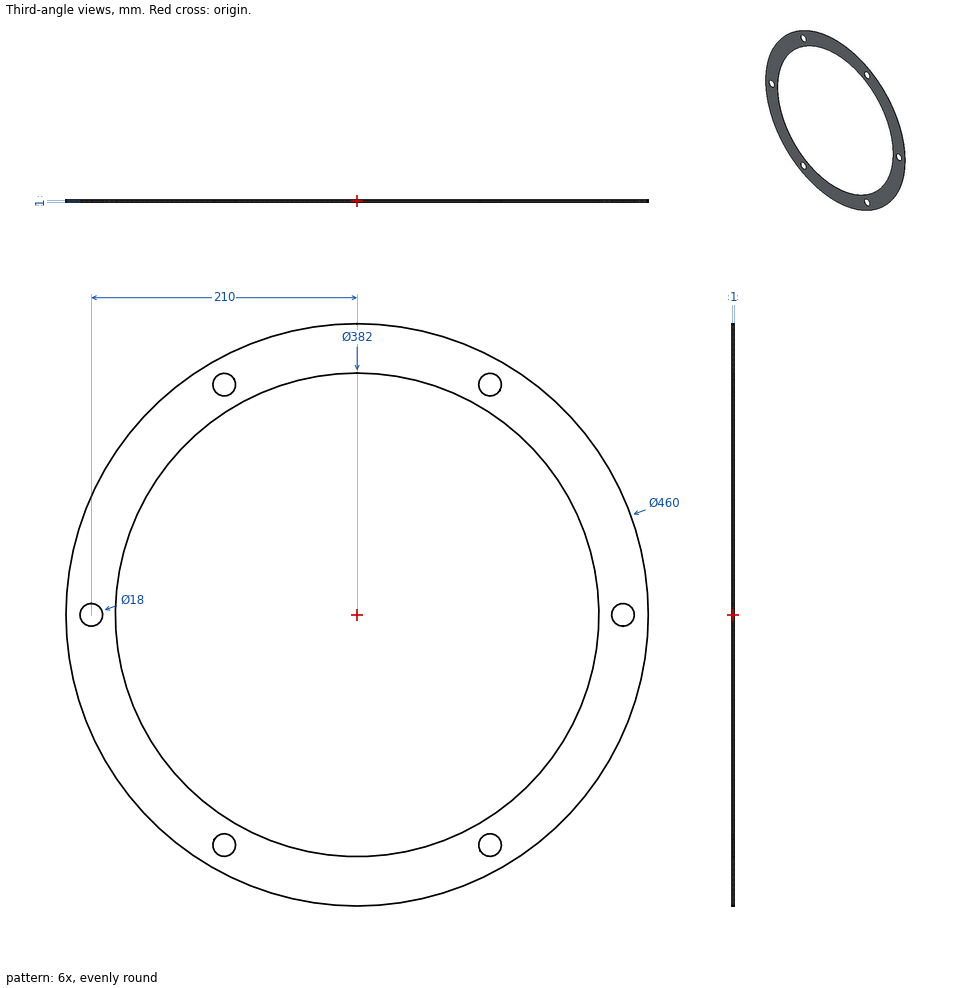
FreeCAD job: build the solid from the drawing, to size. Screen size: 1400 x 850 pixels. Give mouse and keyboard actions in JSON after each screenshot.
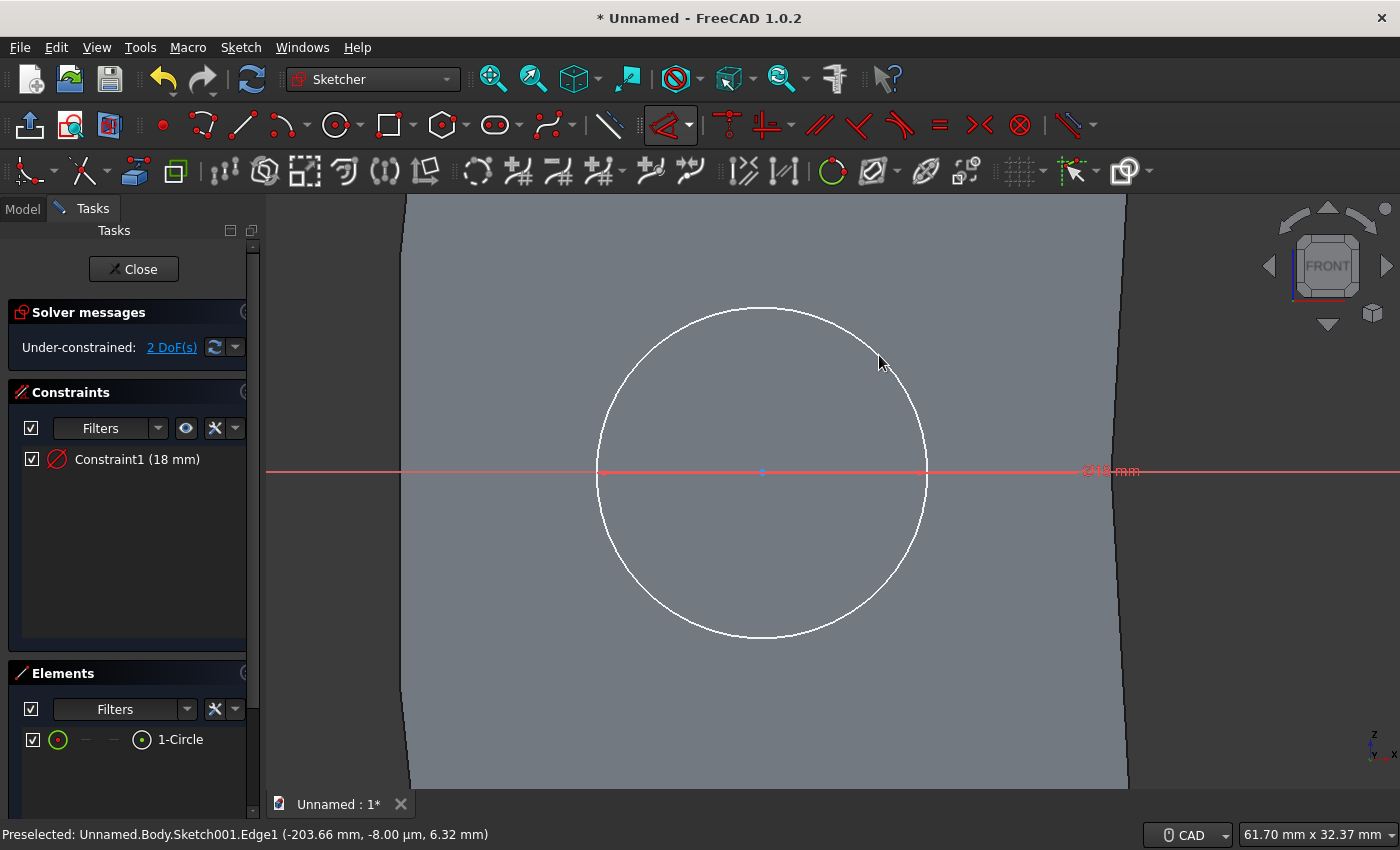
{"action": "left_click", "coordinate": [762, 473]}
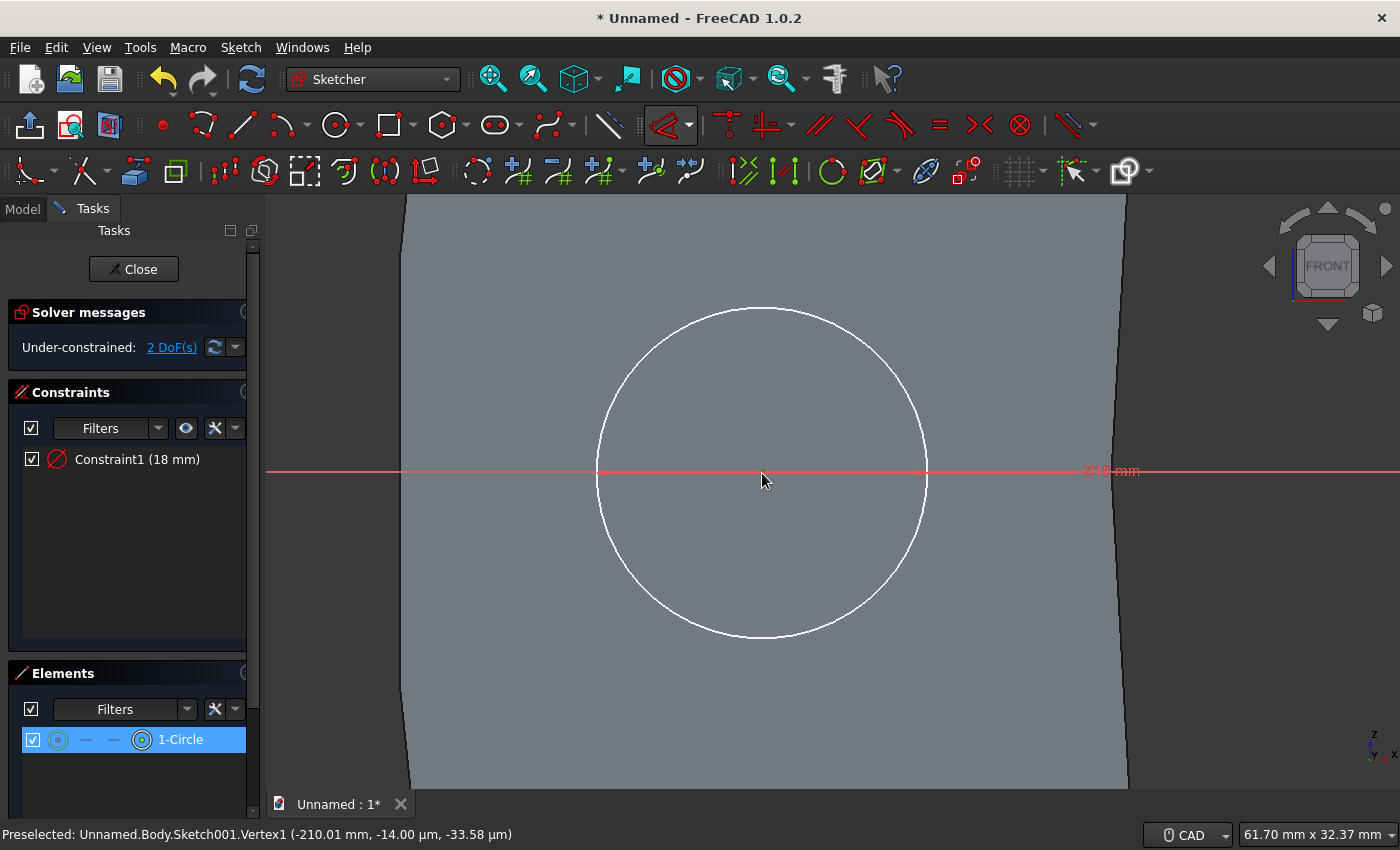
{"action": "left_click", "coordinate": [361, 472]}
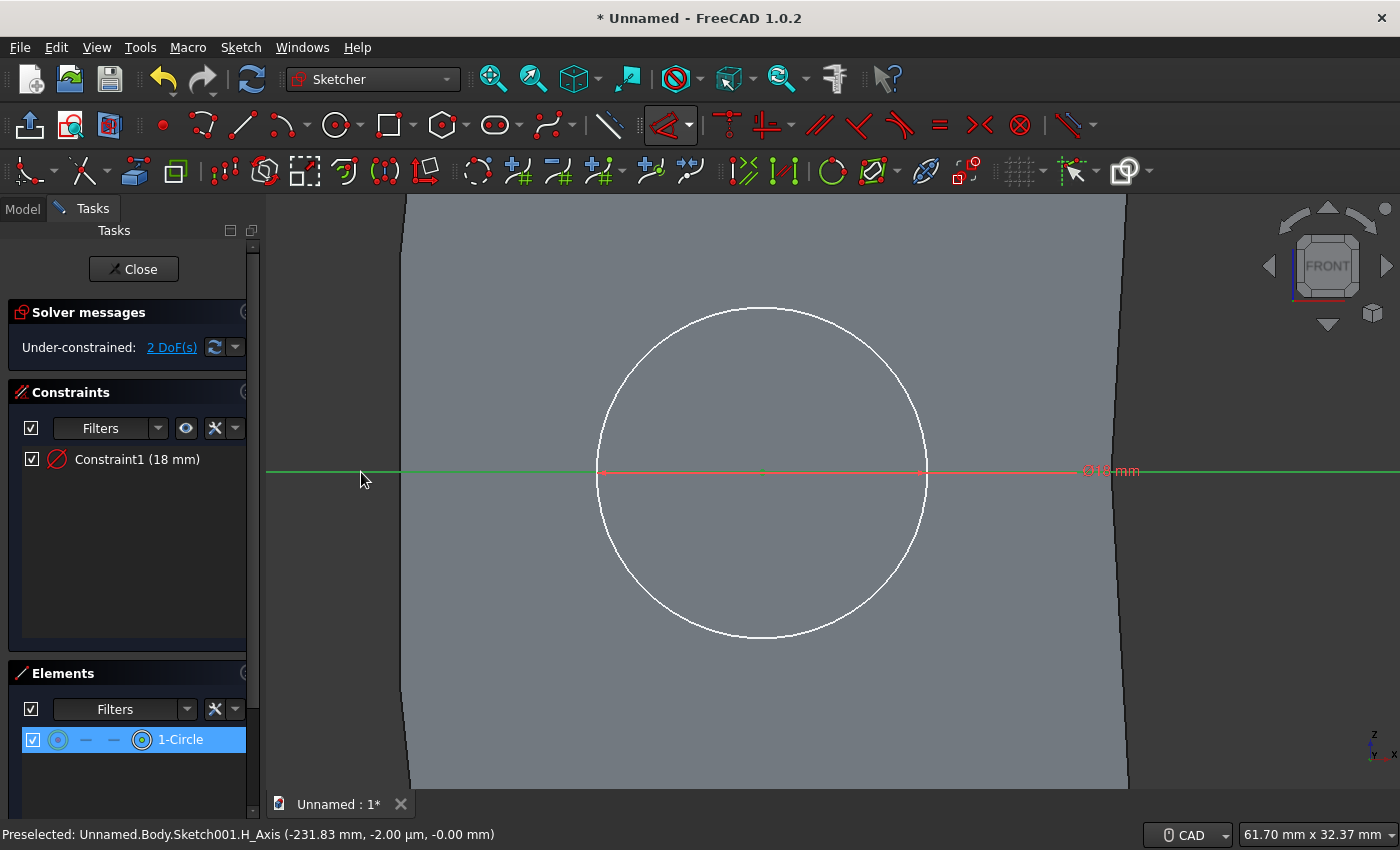
{"action": "left_click", "coordinate": [728, 126]}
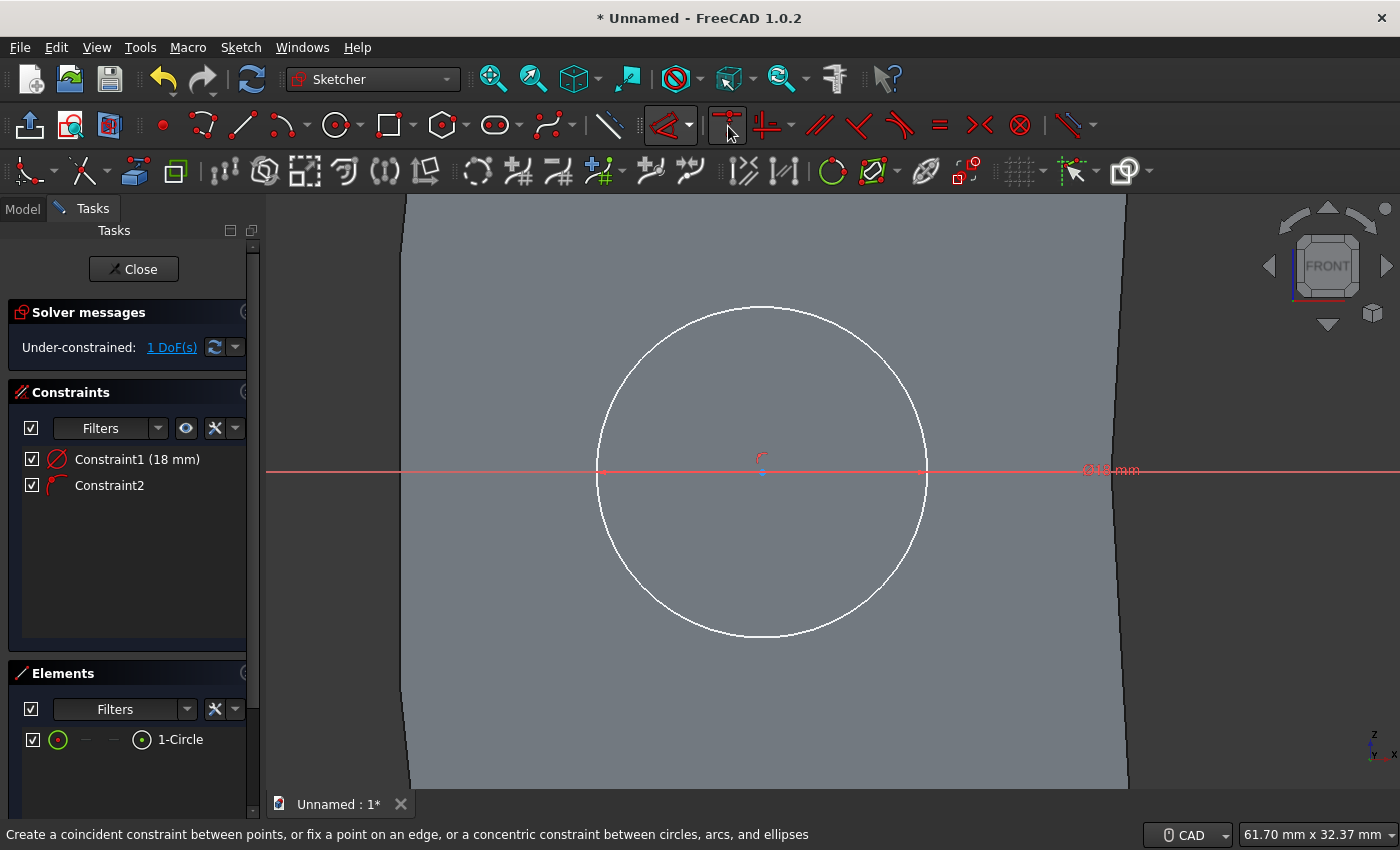
{"action": "left_click", "coordinate": [762, 472]}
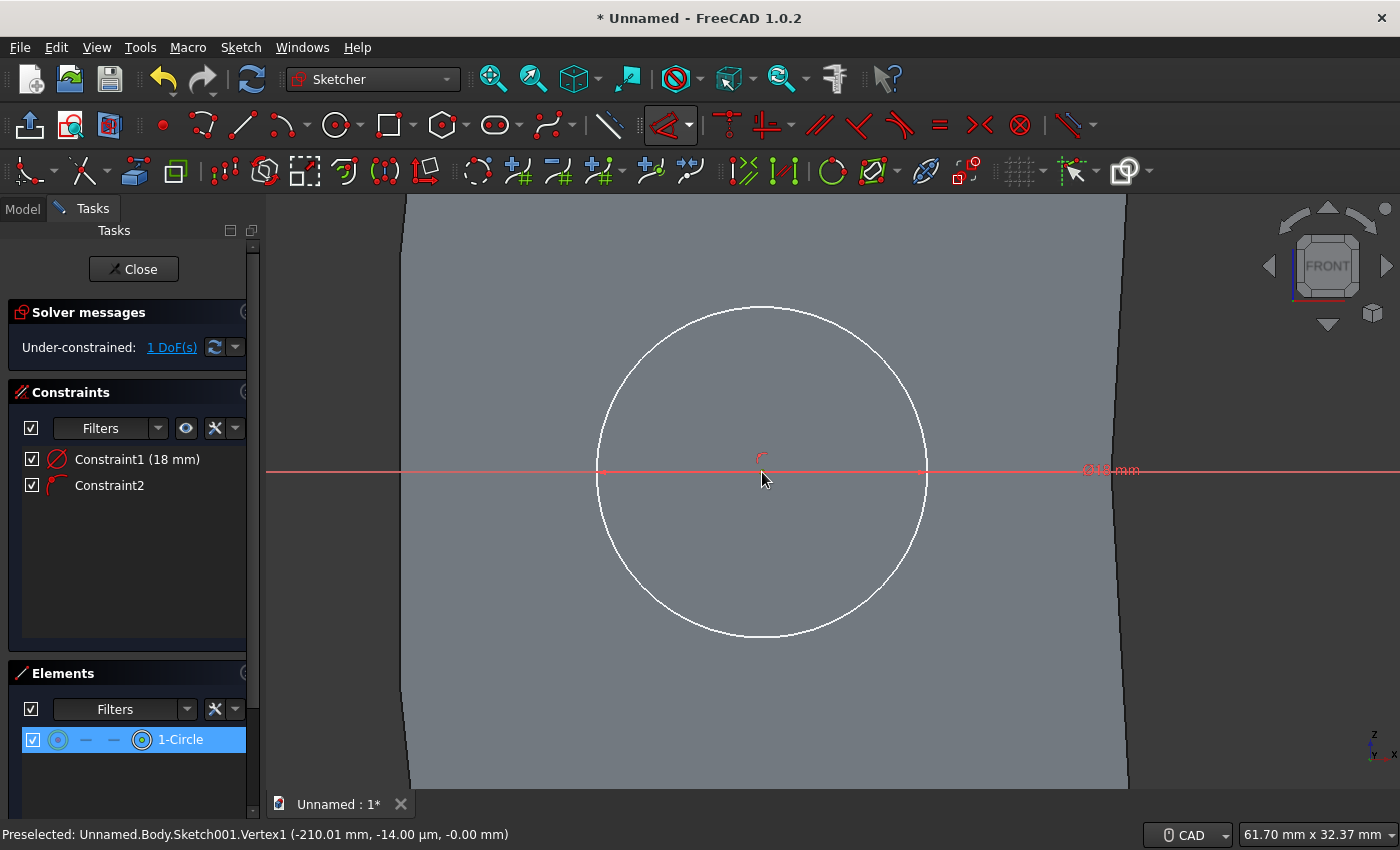
{"action": "key", "text": "l"}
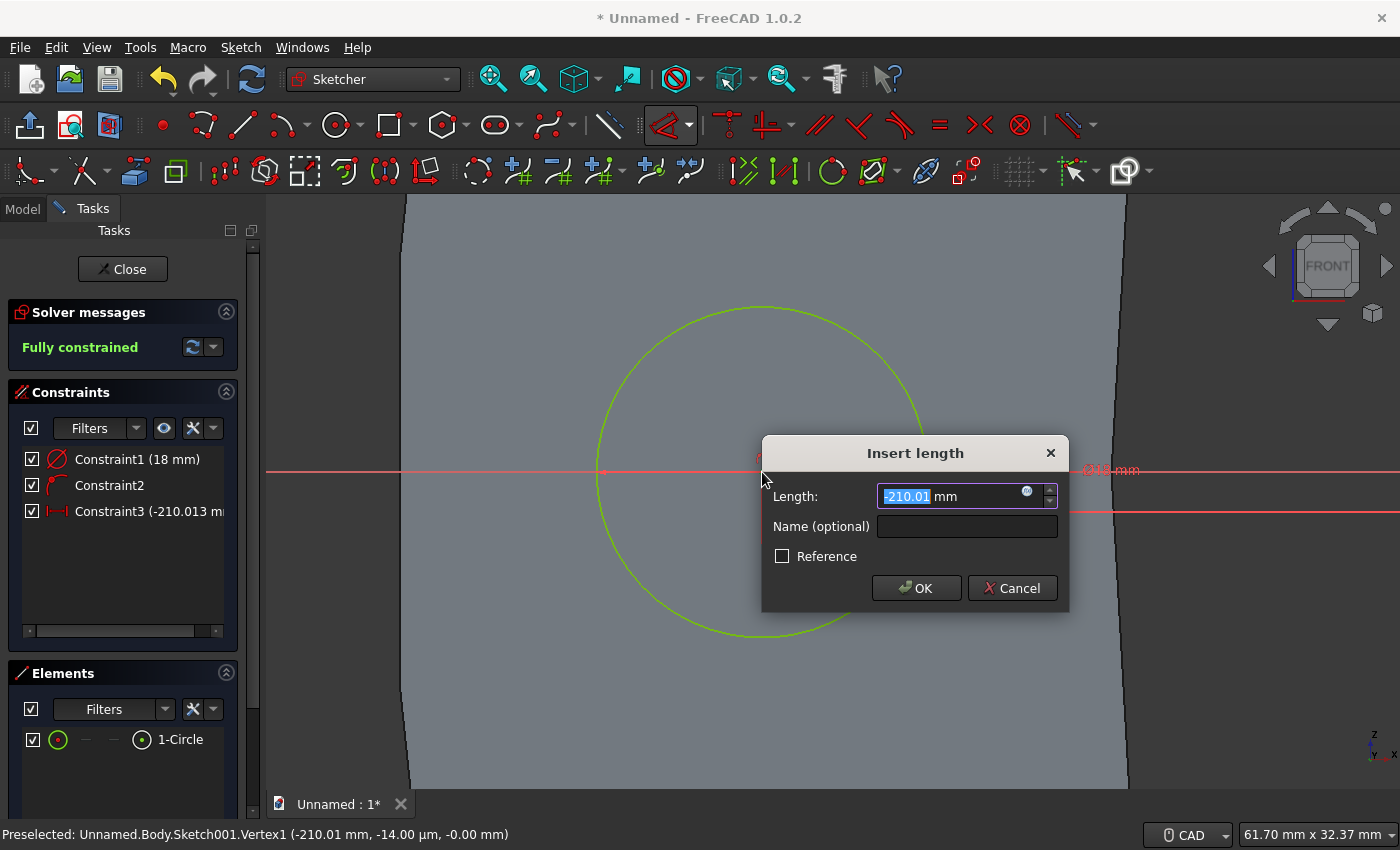
{"action": "type", "text": "-210"}
{"action": "key", "text": "Return"}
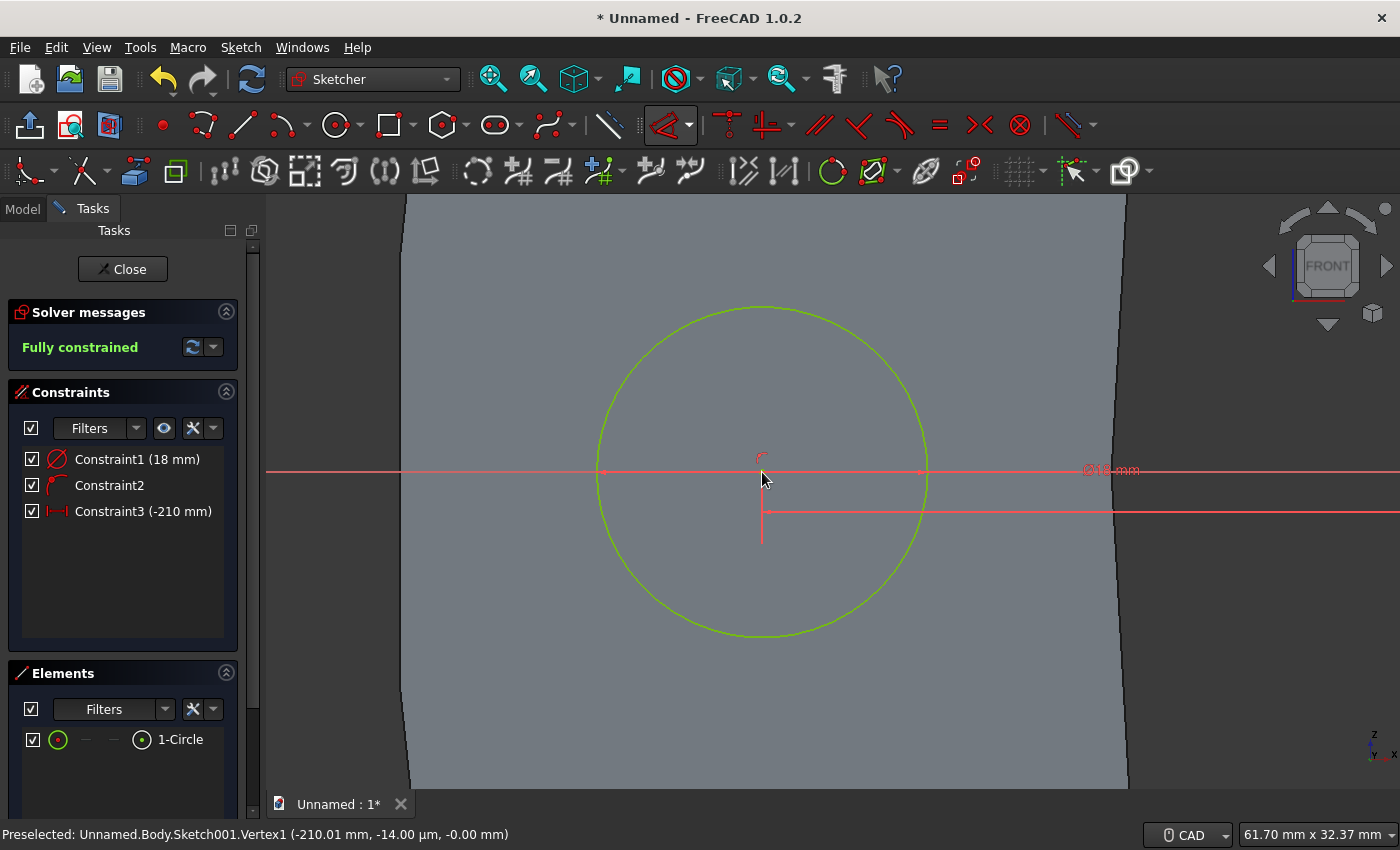
{"action": "left_click", "coordinate": [123, 269]}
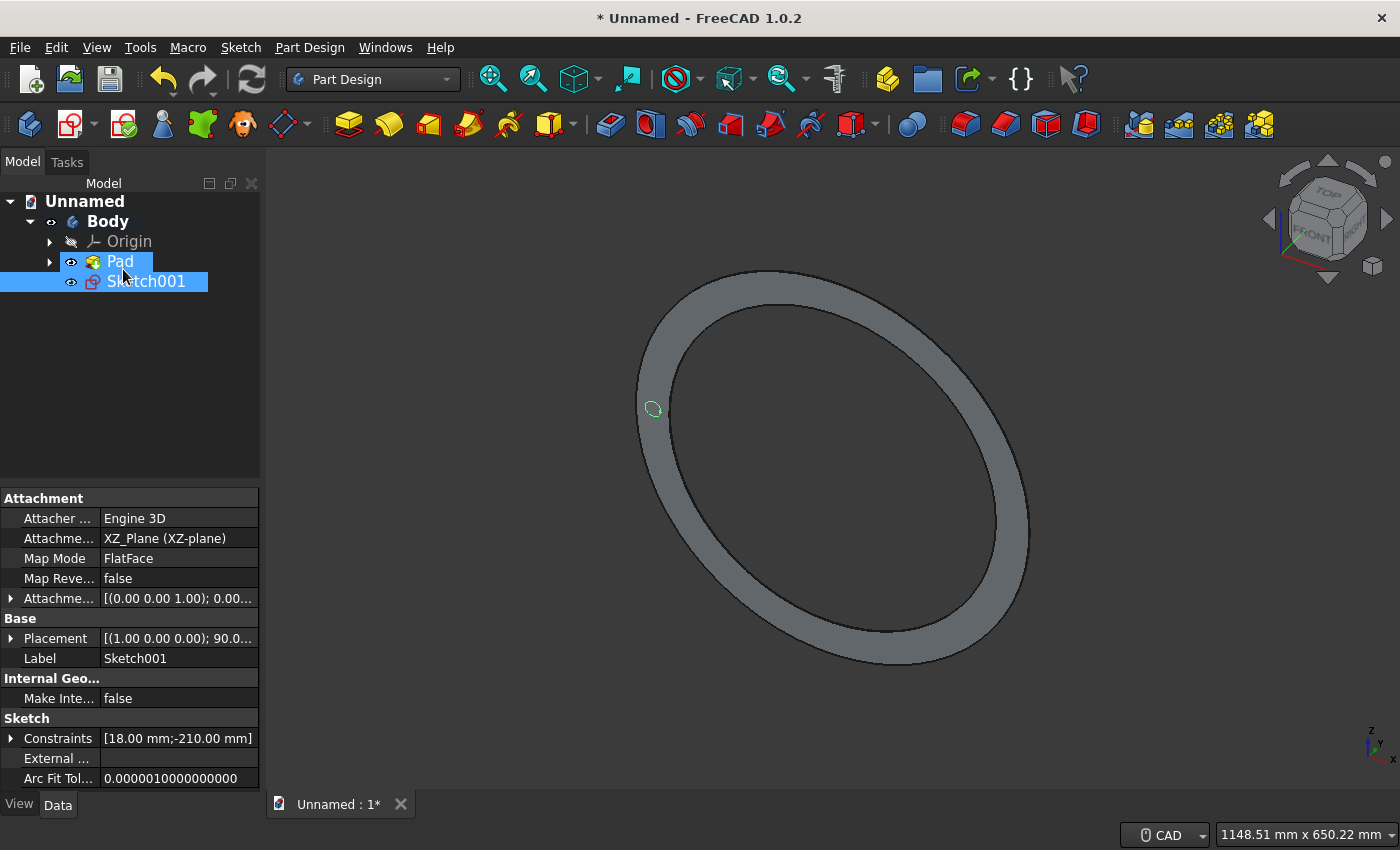
{"action": "left_click", "coordinate": [612, 124]}